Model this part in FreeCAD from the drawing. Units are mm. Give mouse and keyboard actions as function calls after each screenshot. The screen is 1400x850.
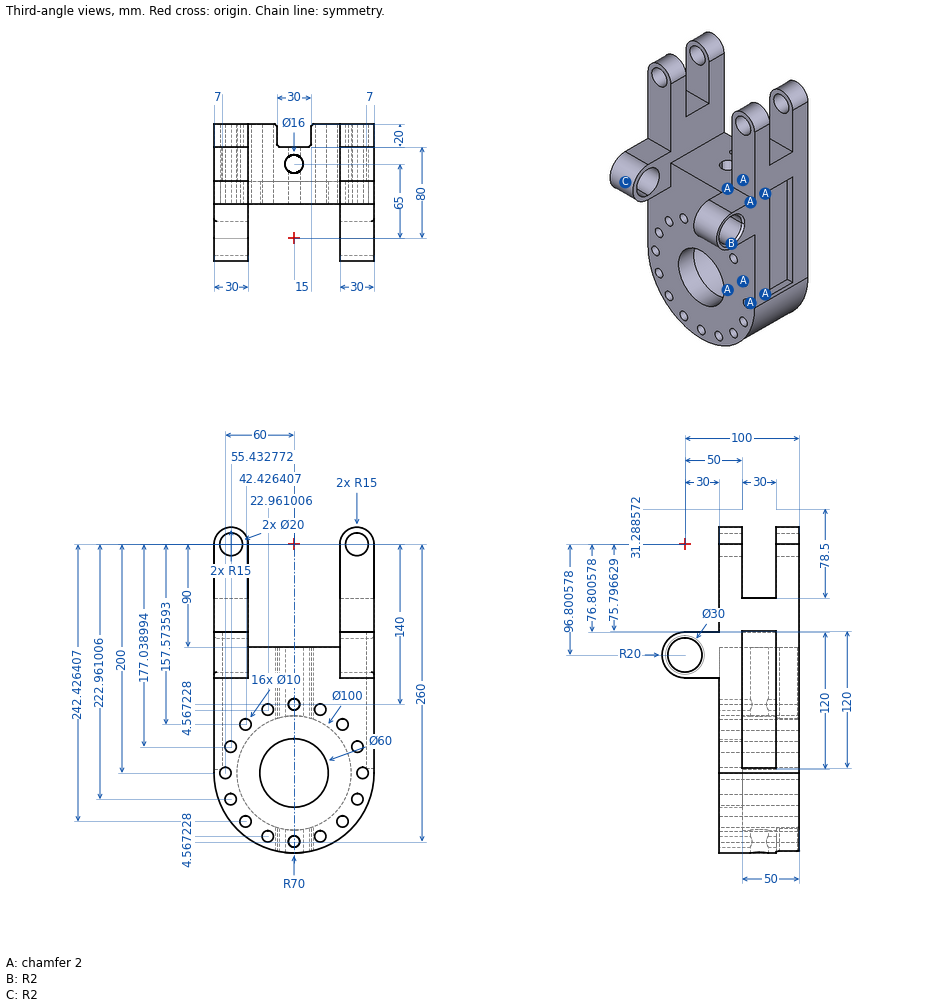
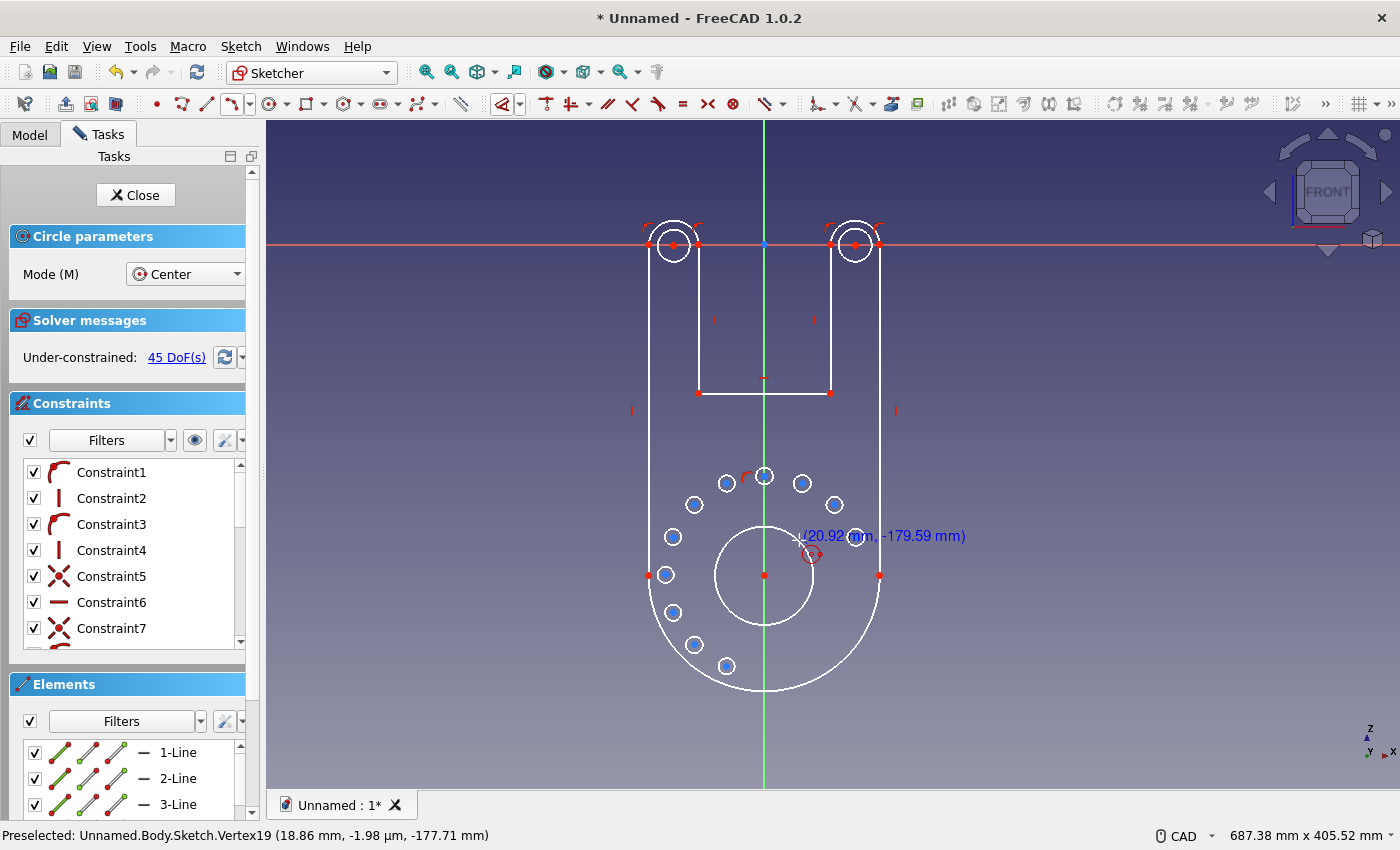
scroll(764, 674, up, 6)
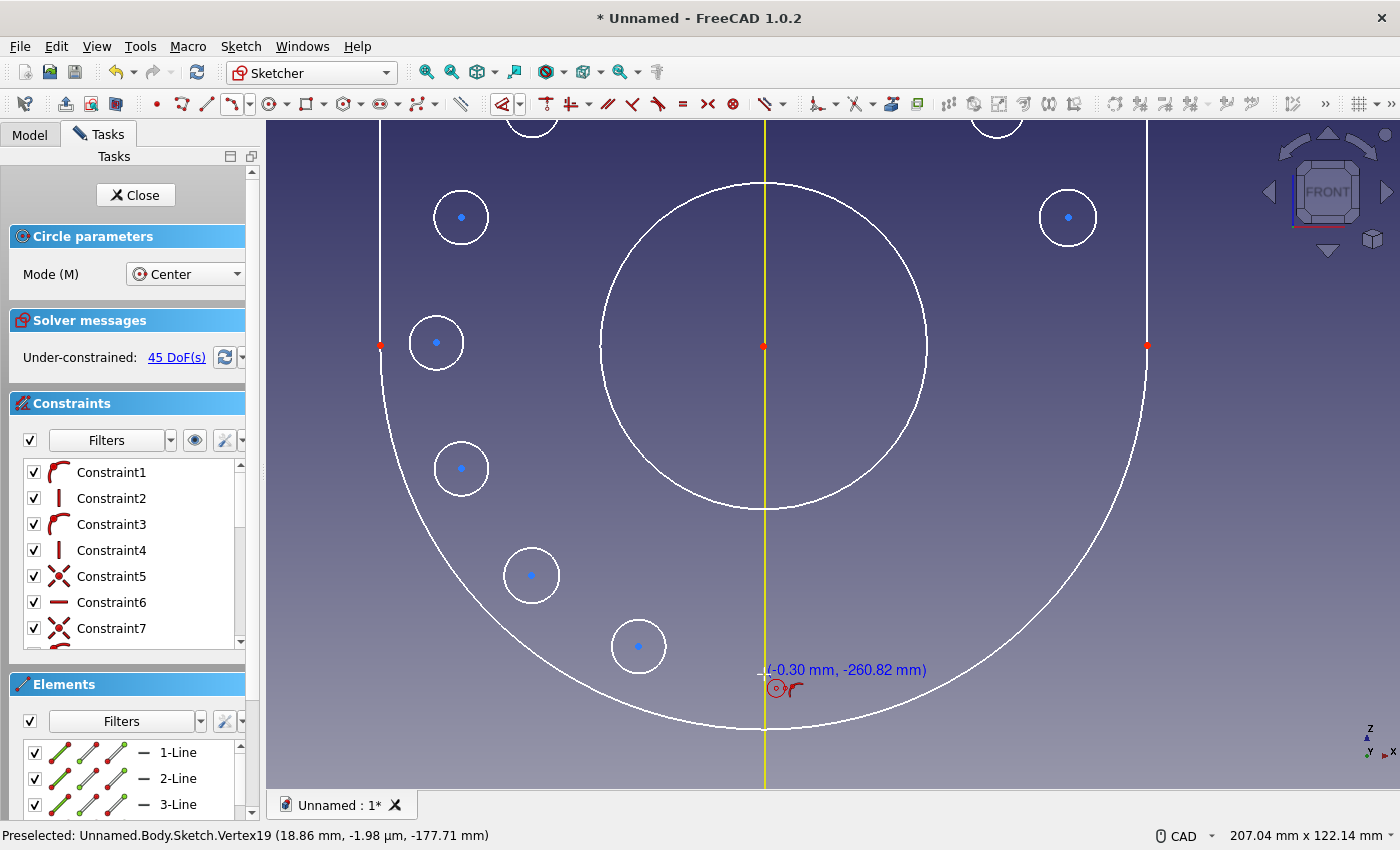
click(765, 671)
click(784, 652)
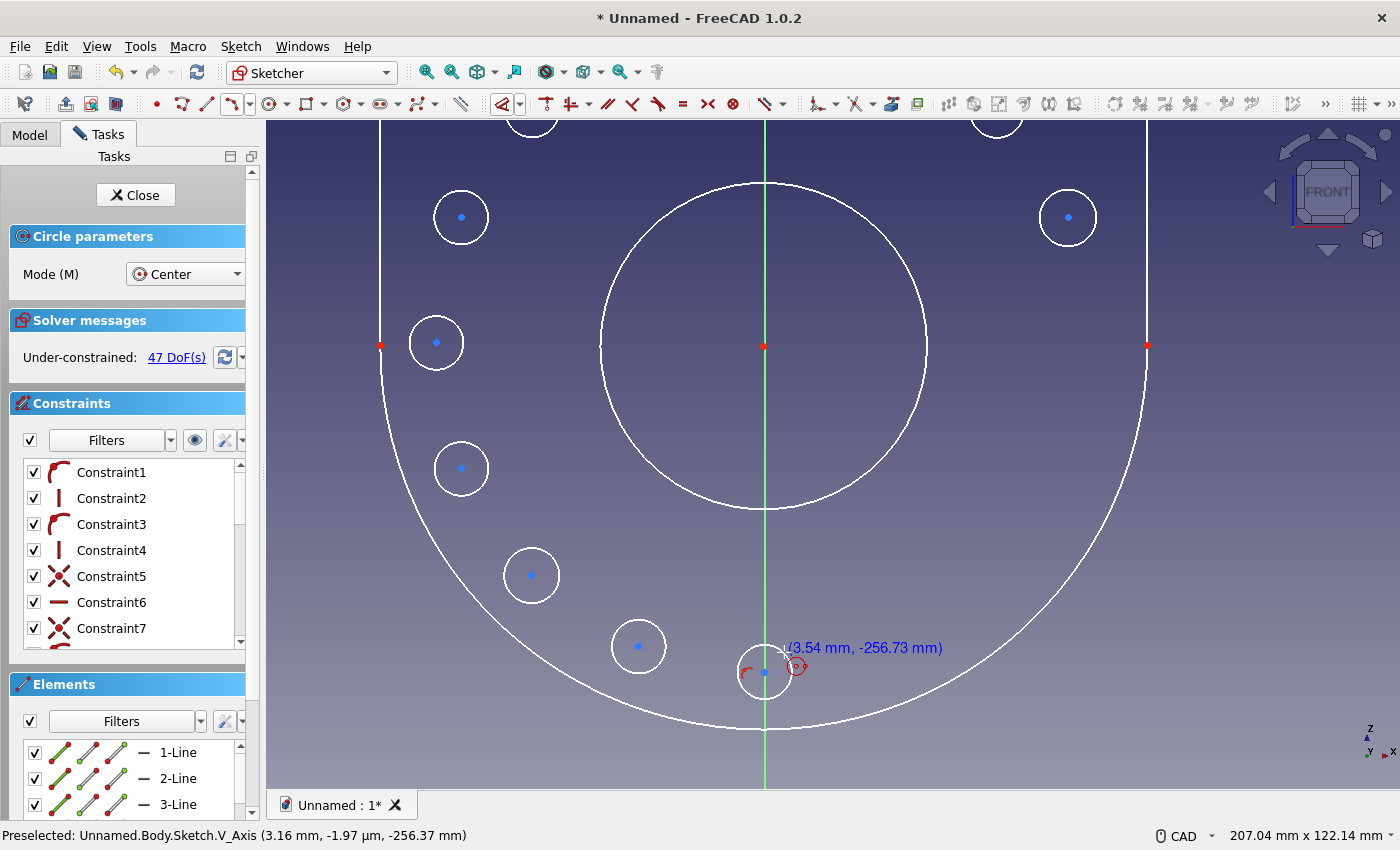
click(890, 646)
click(910, 627)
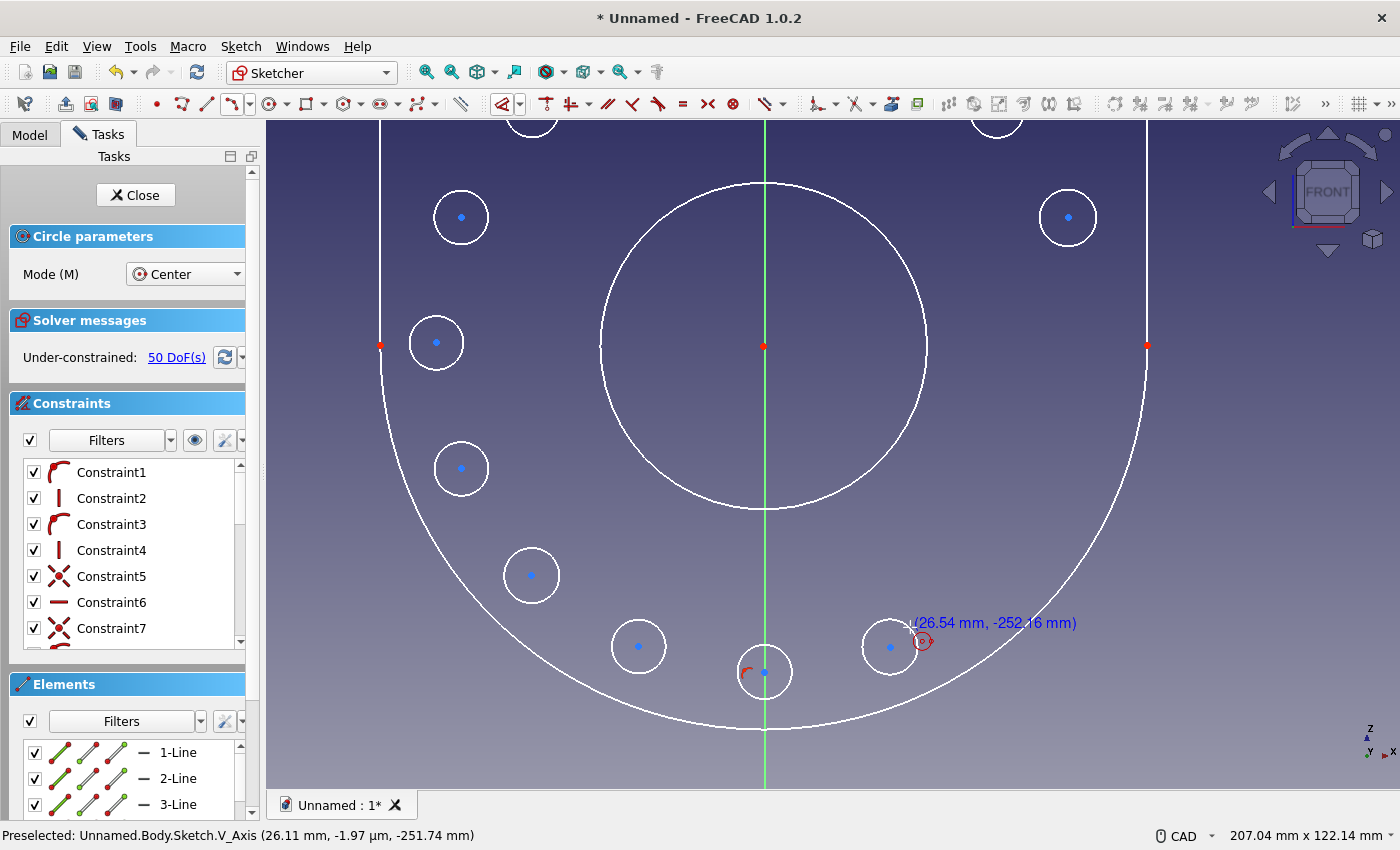
click(1093, 342)
click(1113, 323)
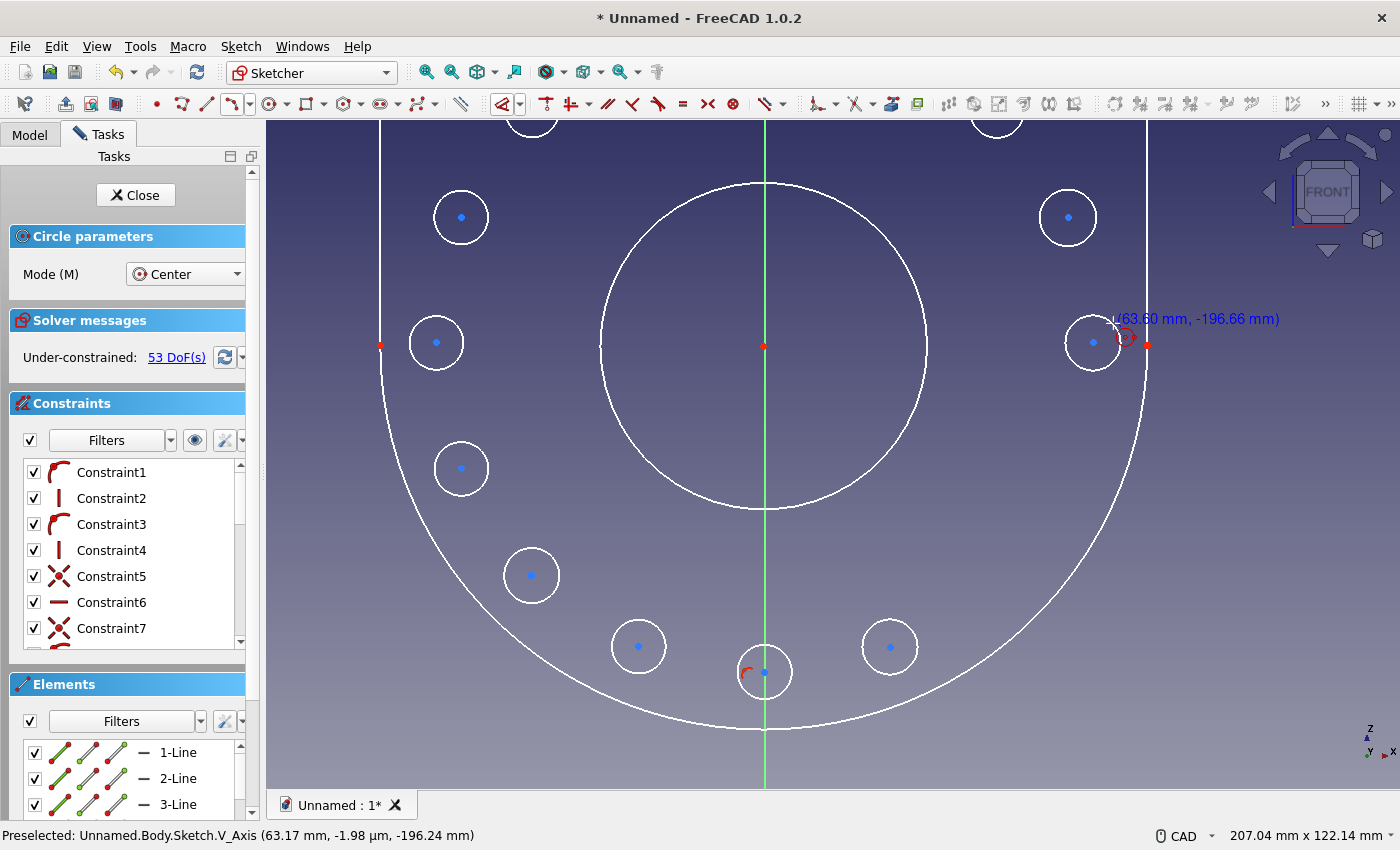
click(1068, 468)
click(1088, 449)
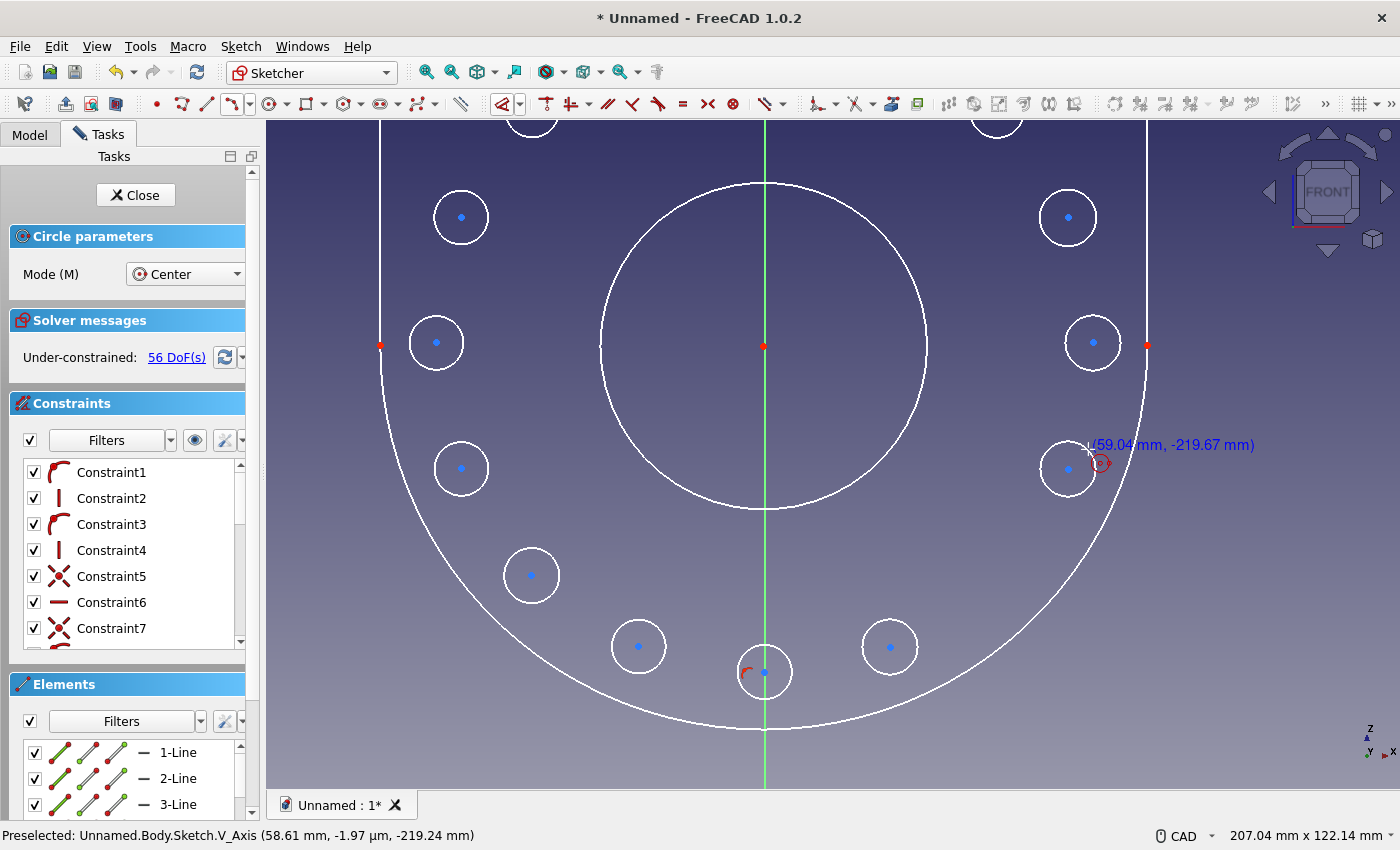
click(997, 575)
click(1016, 555)
key(Escape)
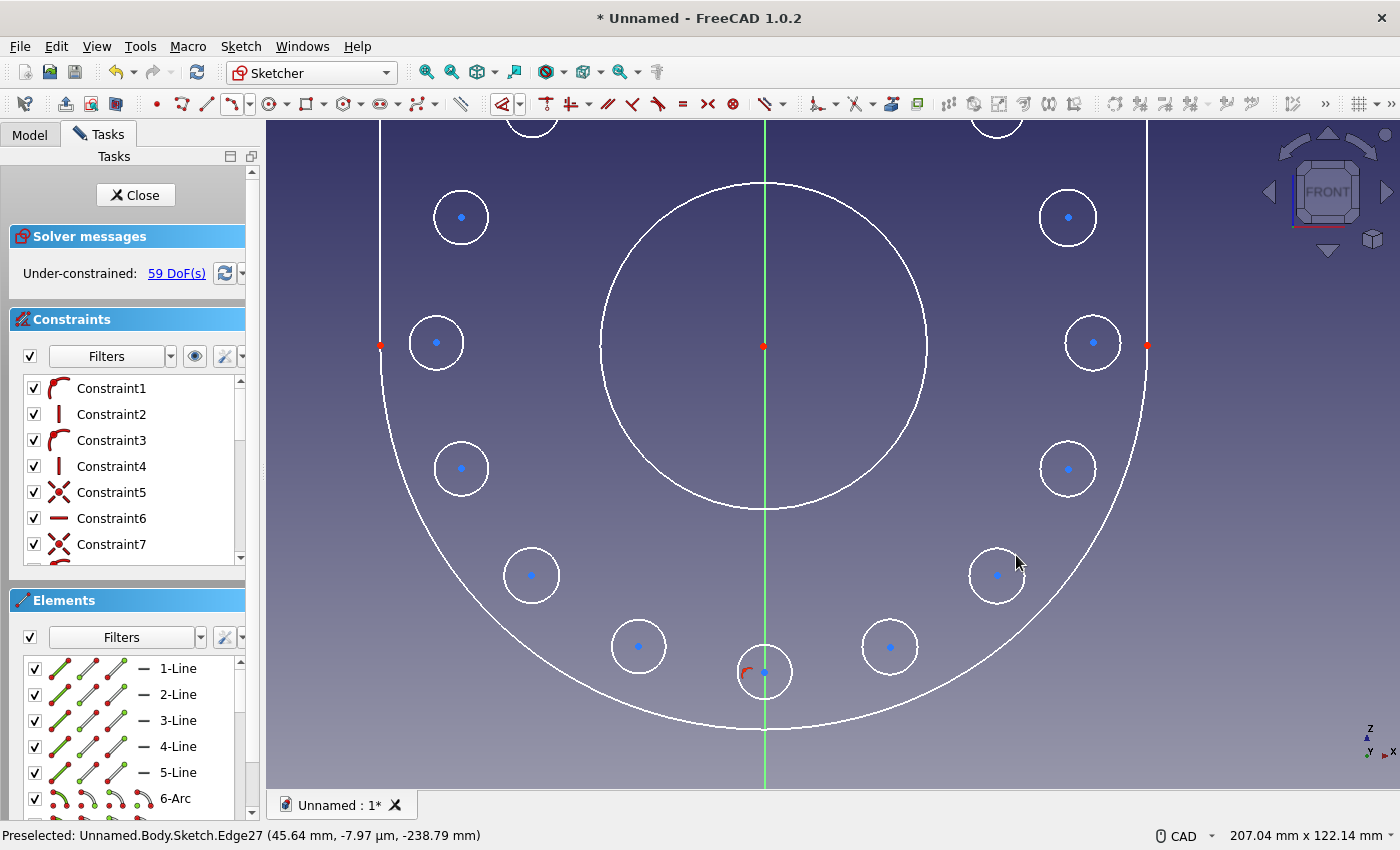
scroll(764, 674, down, 6)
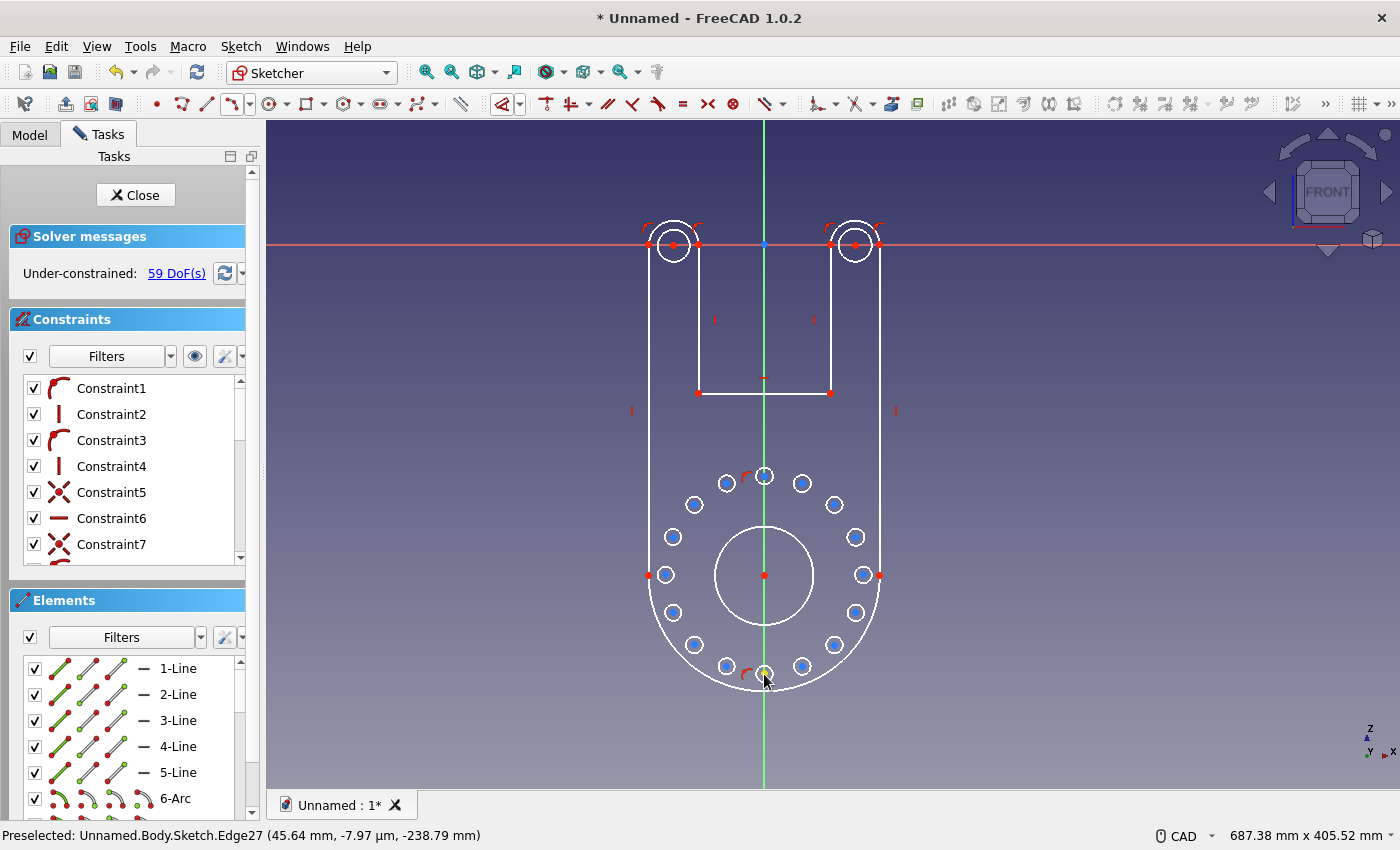
click(649, 476)